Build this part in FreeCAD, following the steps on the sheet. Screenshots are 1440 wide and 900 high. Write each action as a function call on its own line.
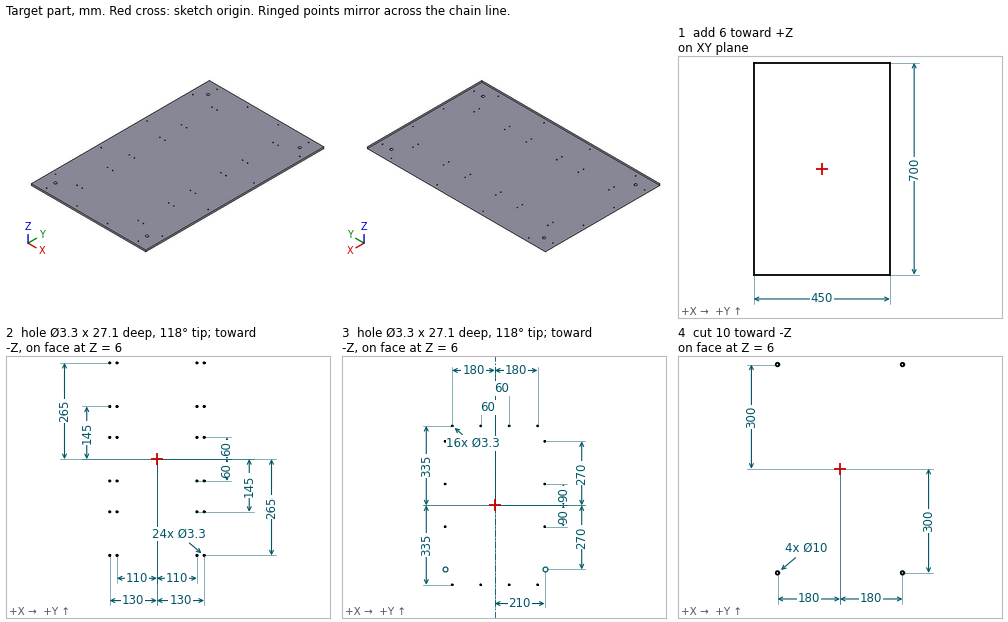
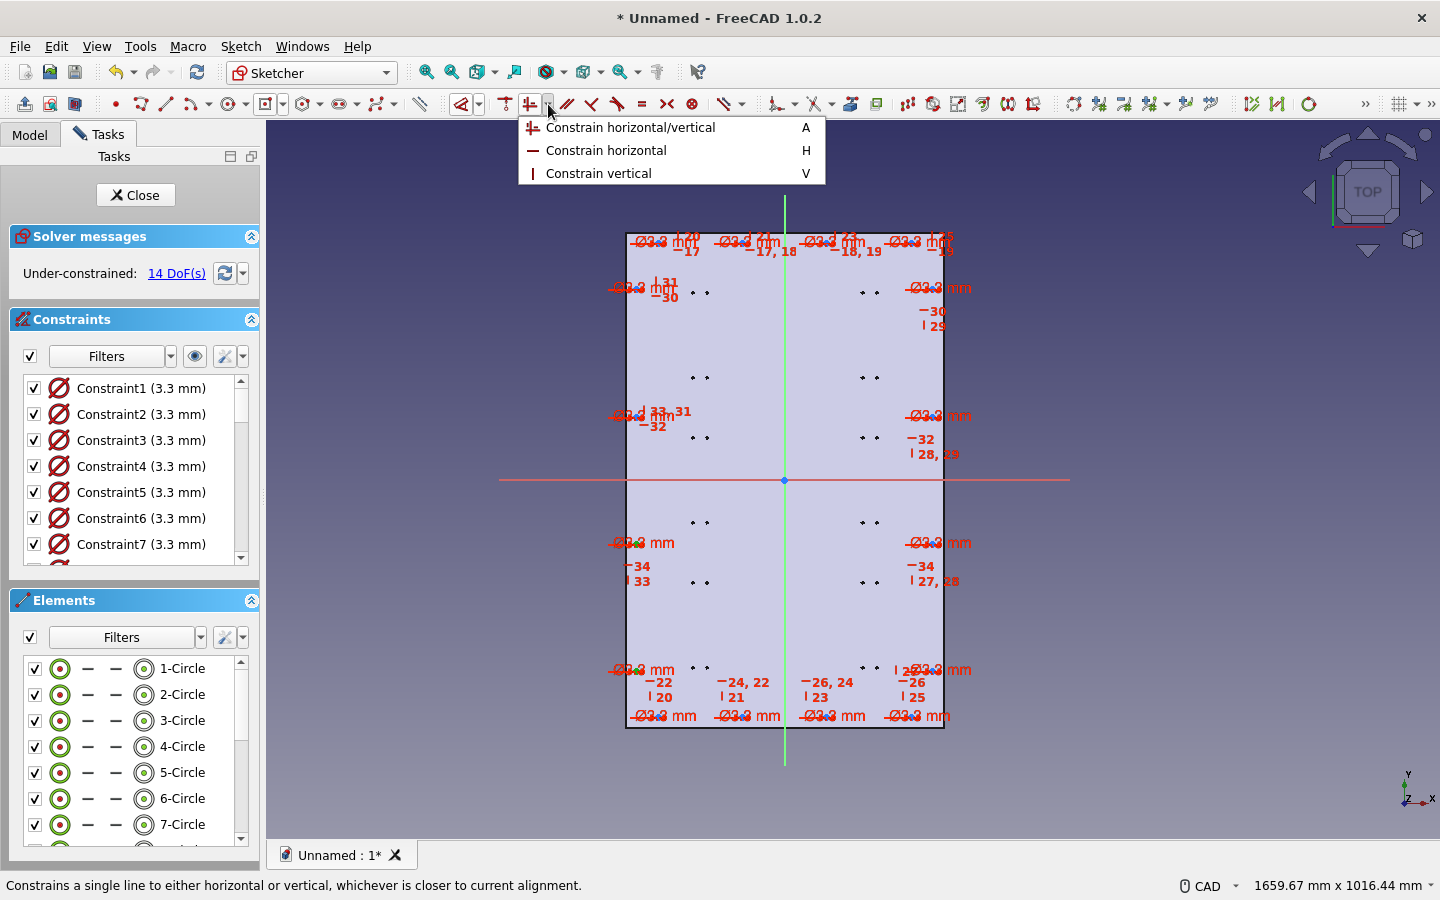
click(672, 174)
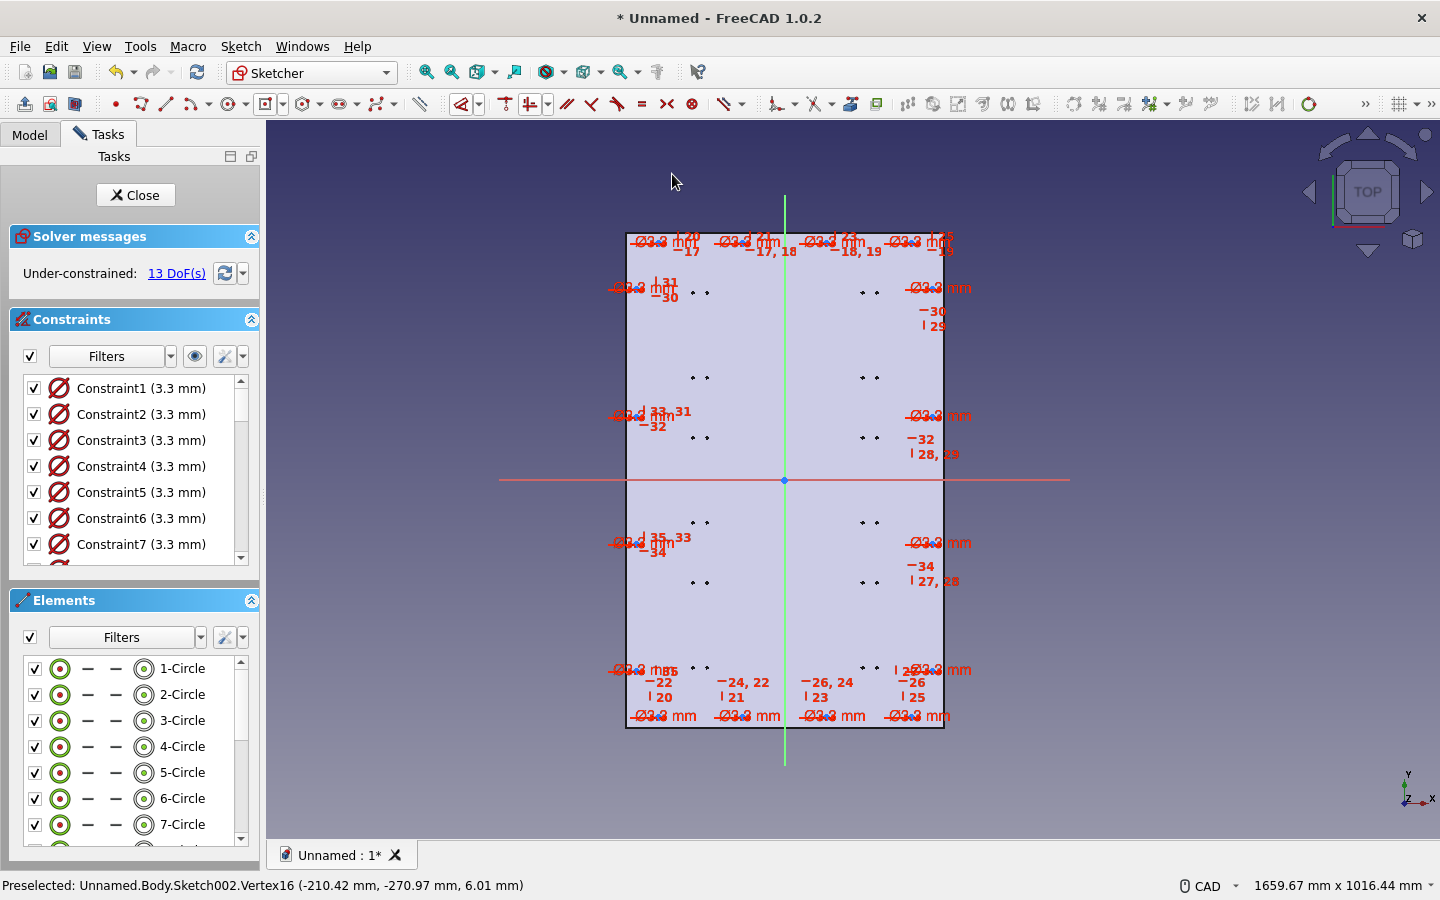
click(933, 672)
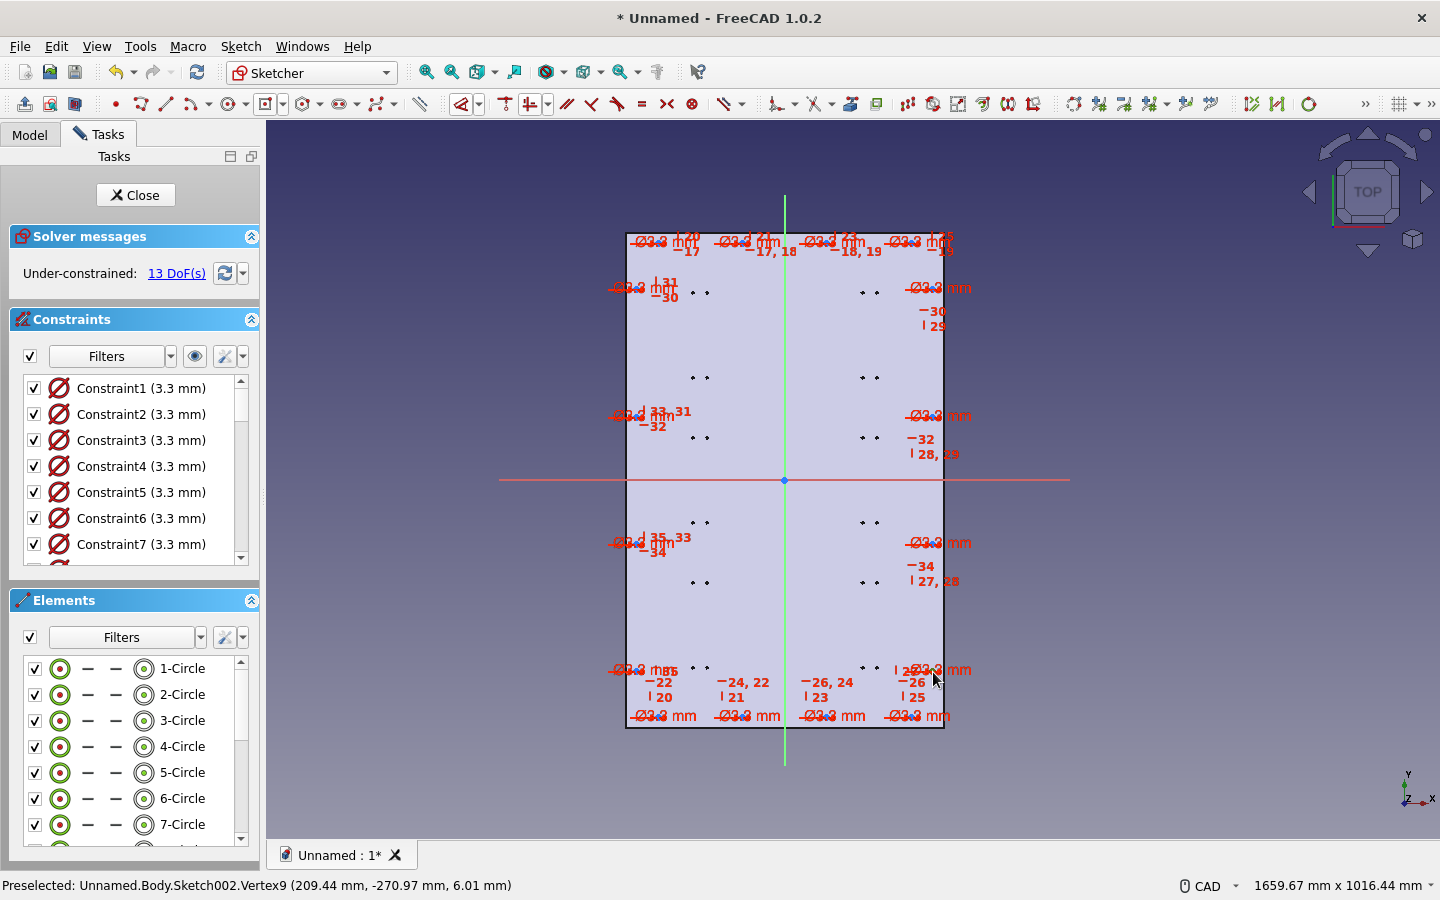
click(636, 672)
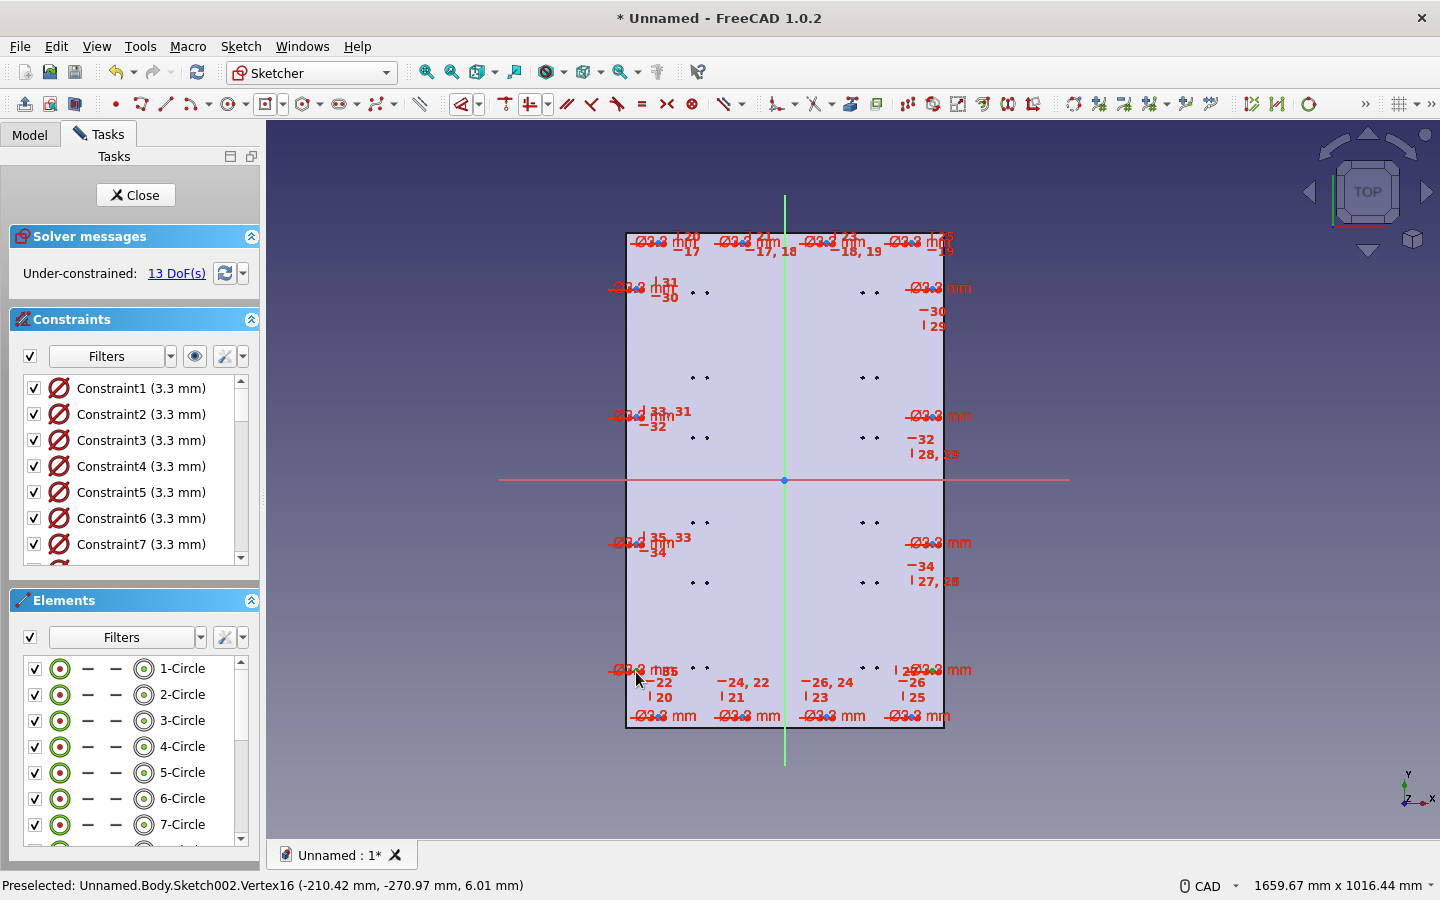
click(785, 764)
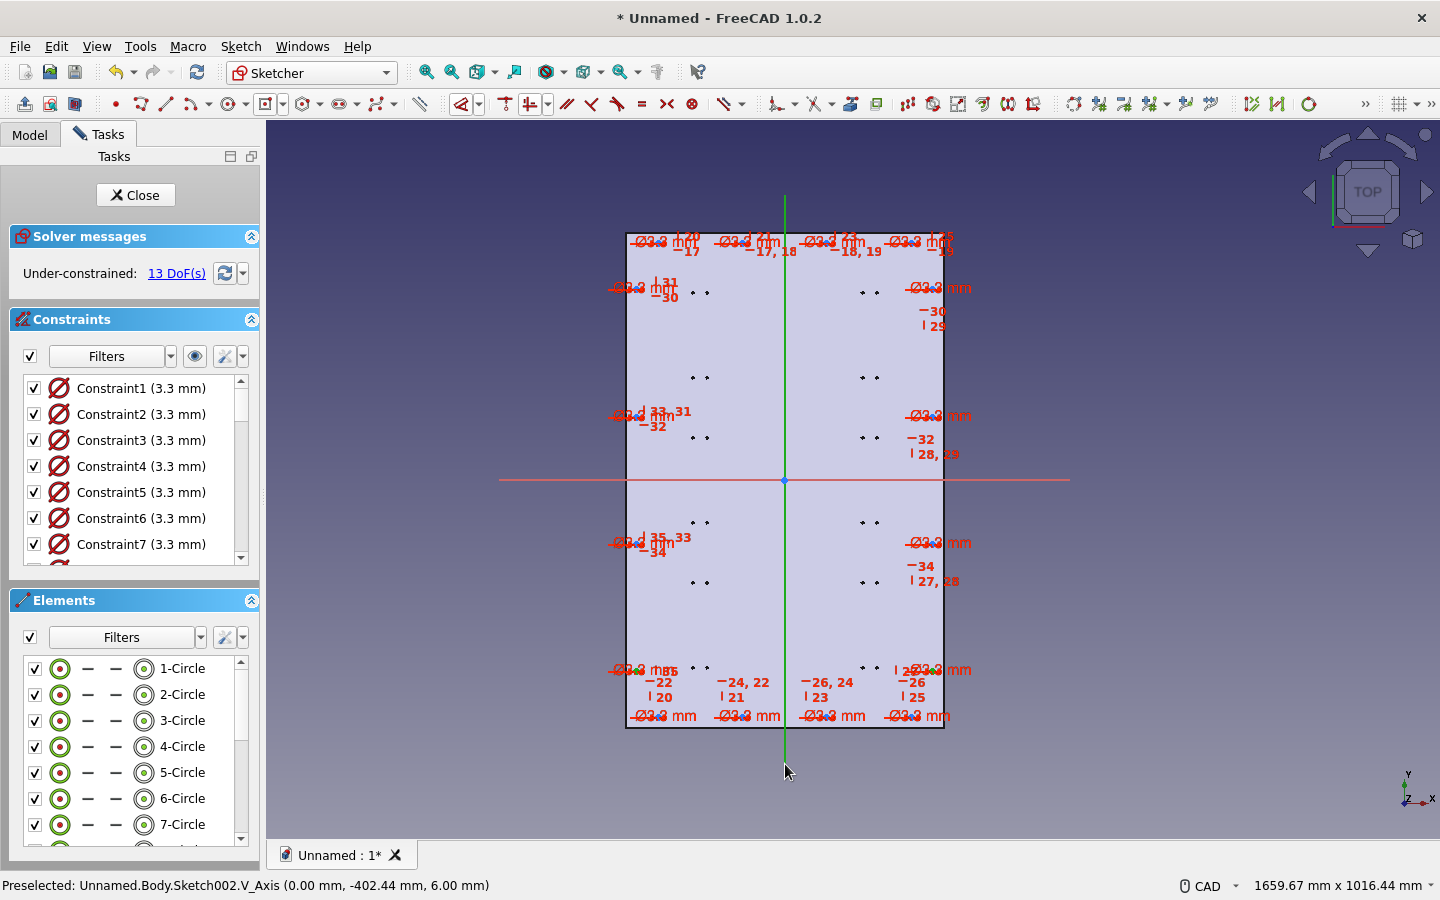
click(667, 104)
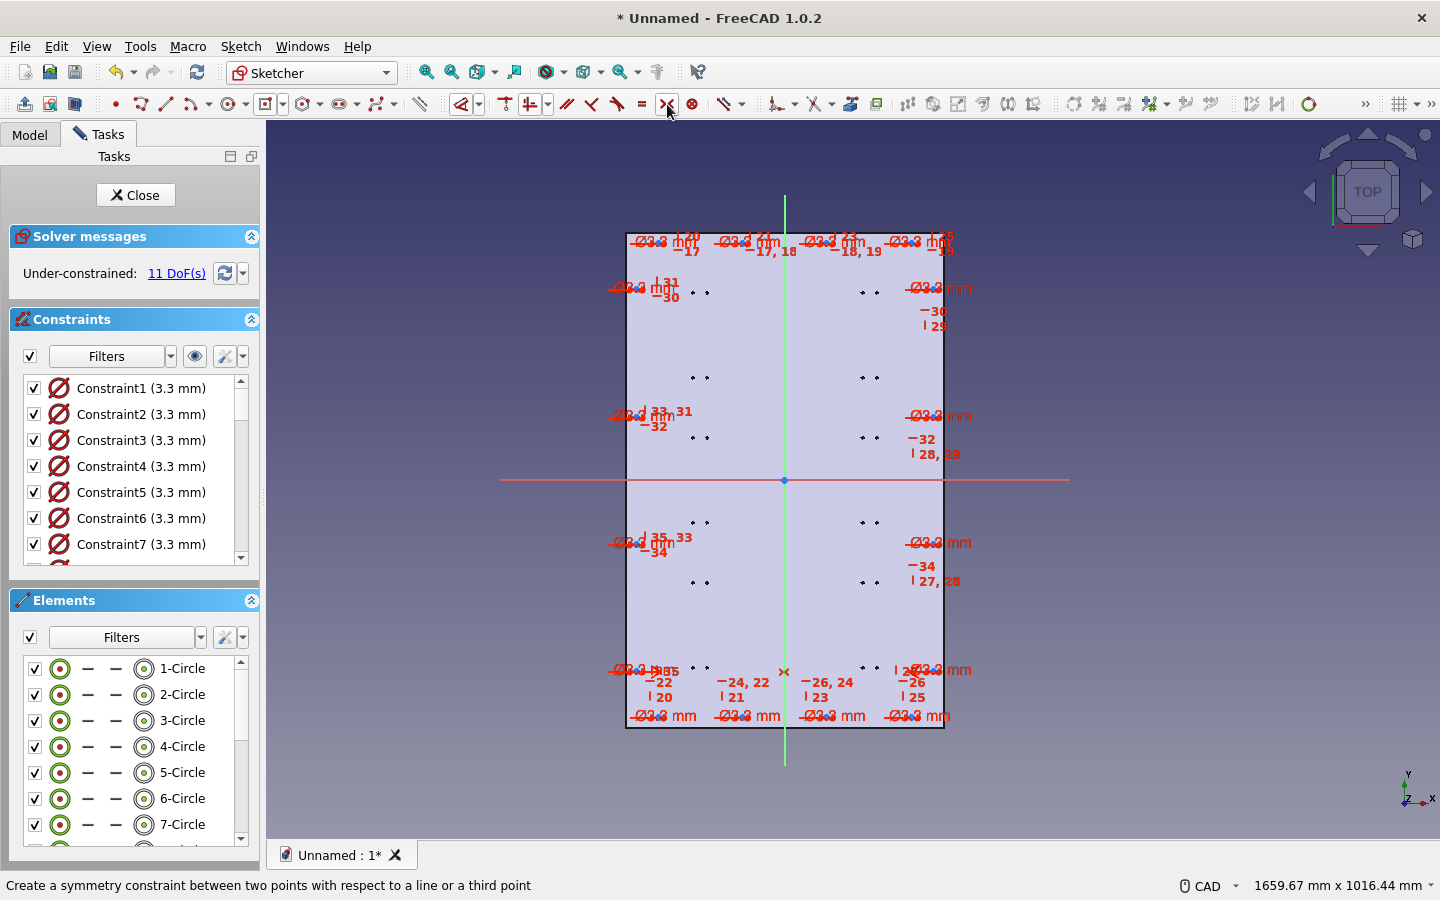
click(742, 244)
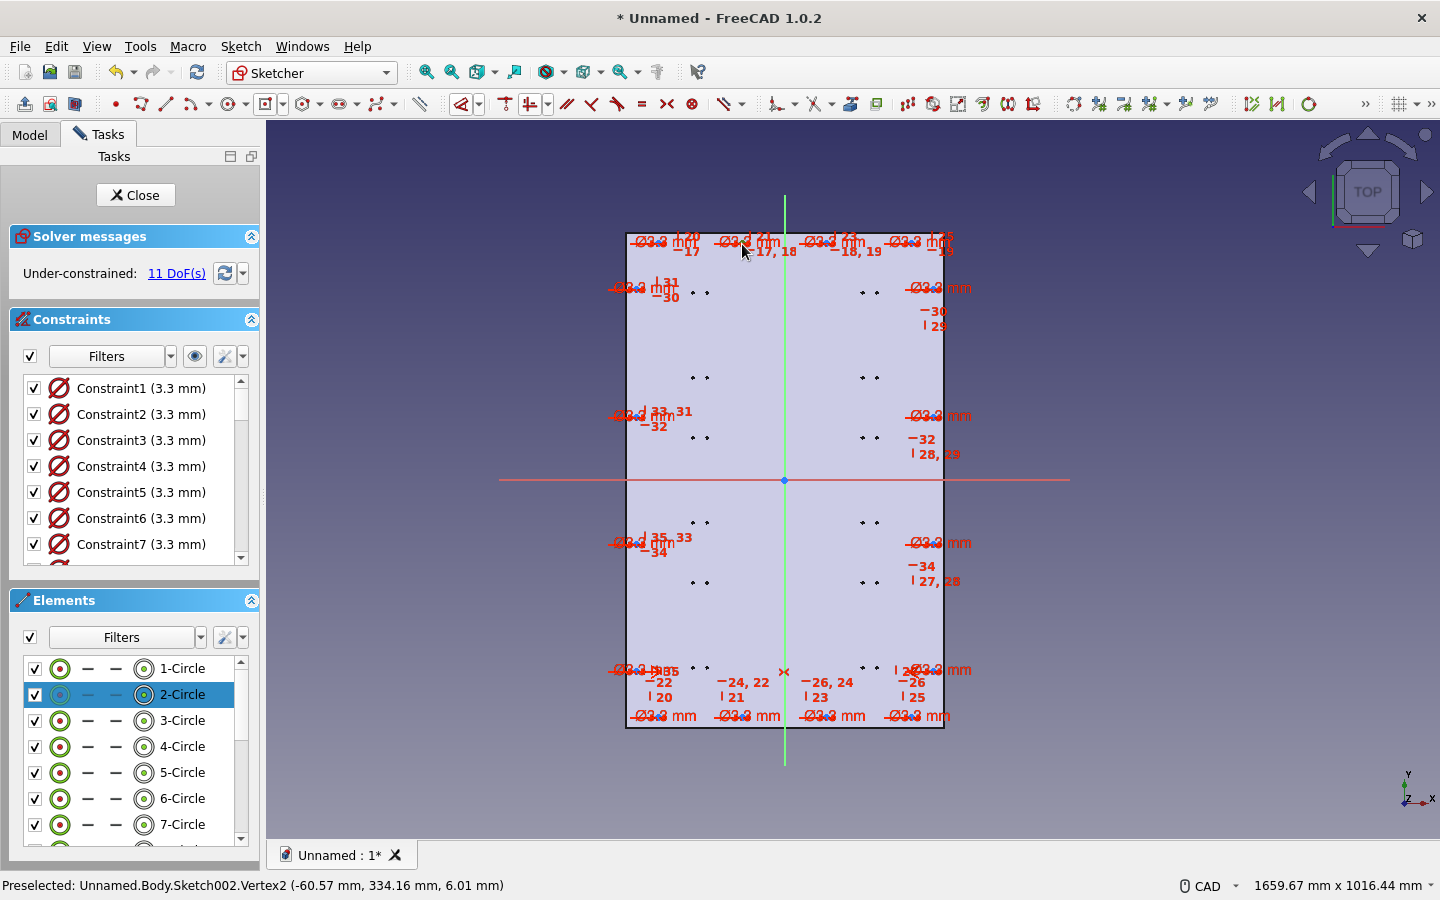
click(478, 104)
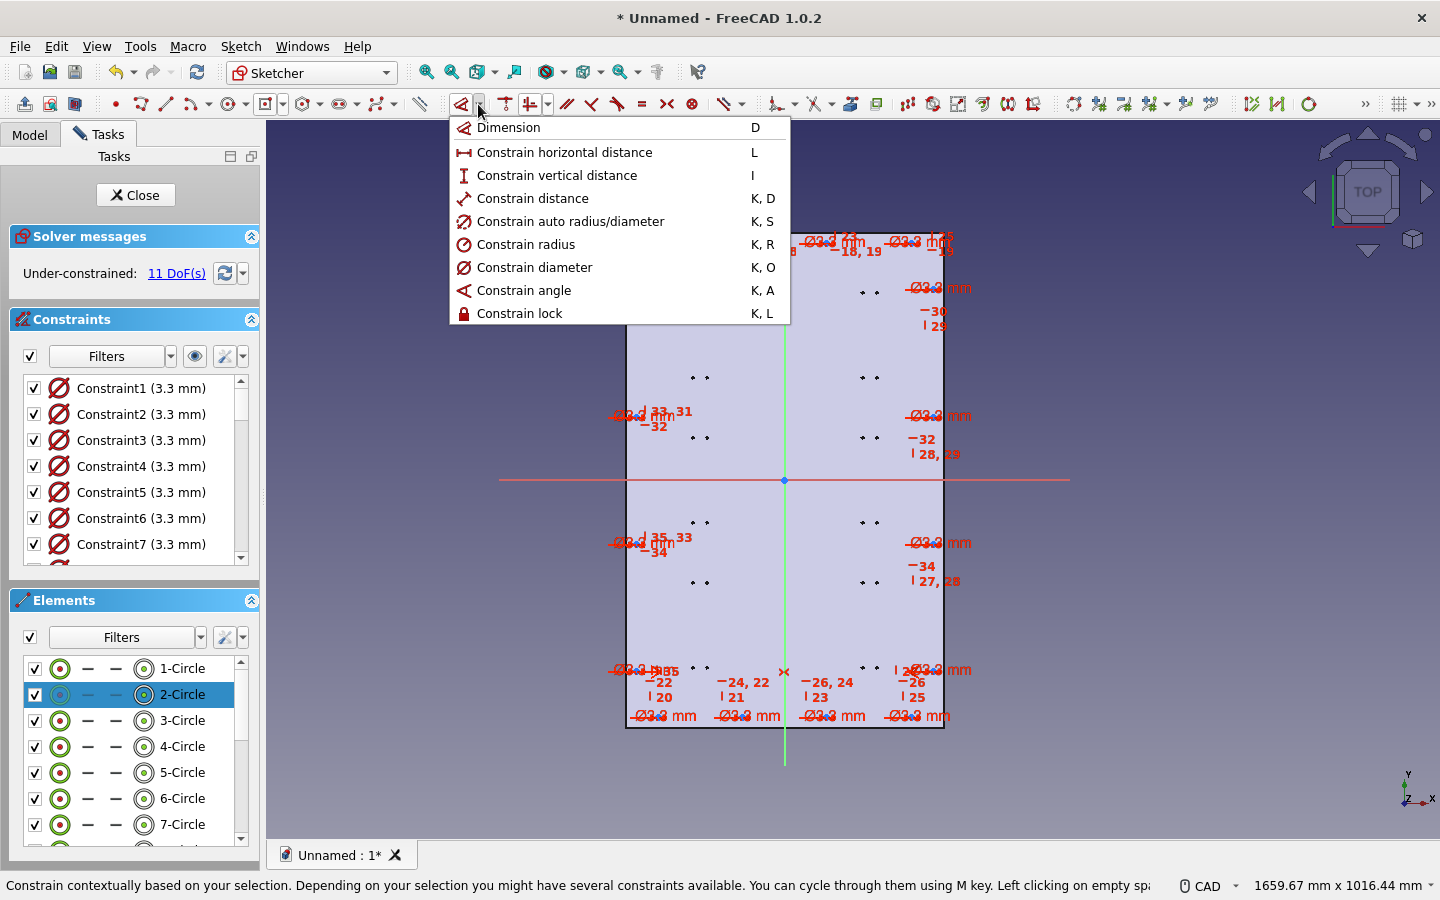
click(620, 152)